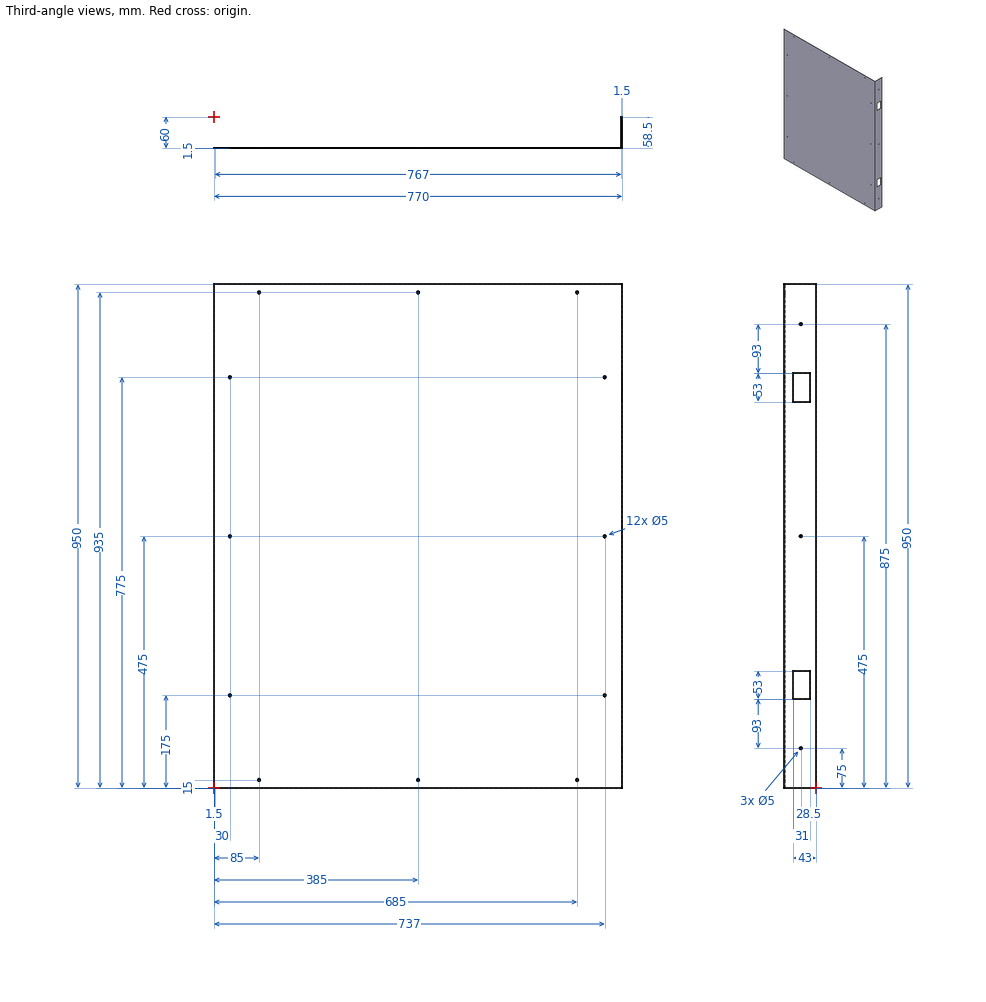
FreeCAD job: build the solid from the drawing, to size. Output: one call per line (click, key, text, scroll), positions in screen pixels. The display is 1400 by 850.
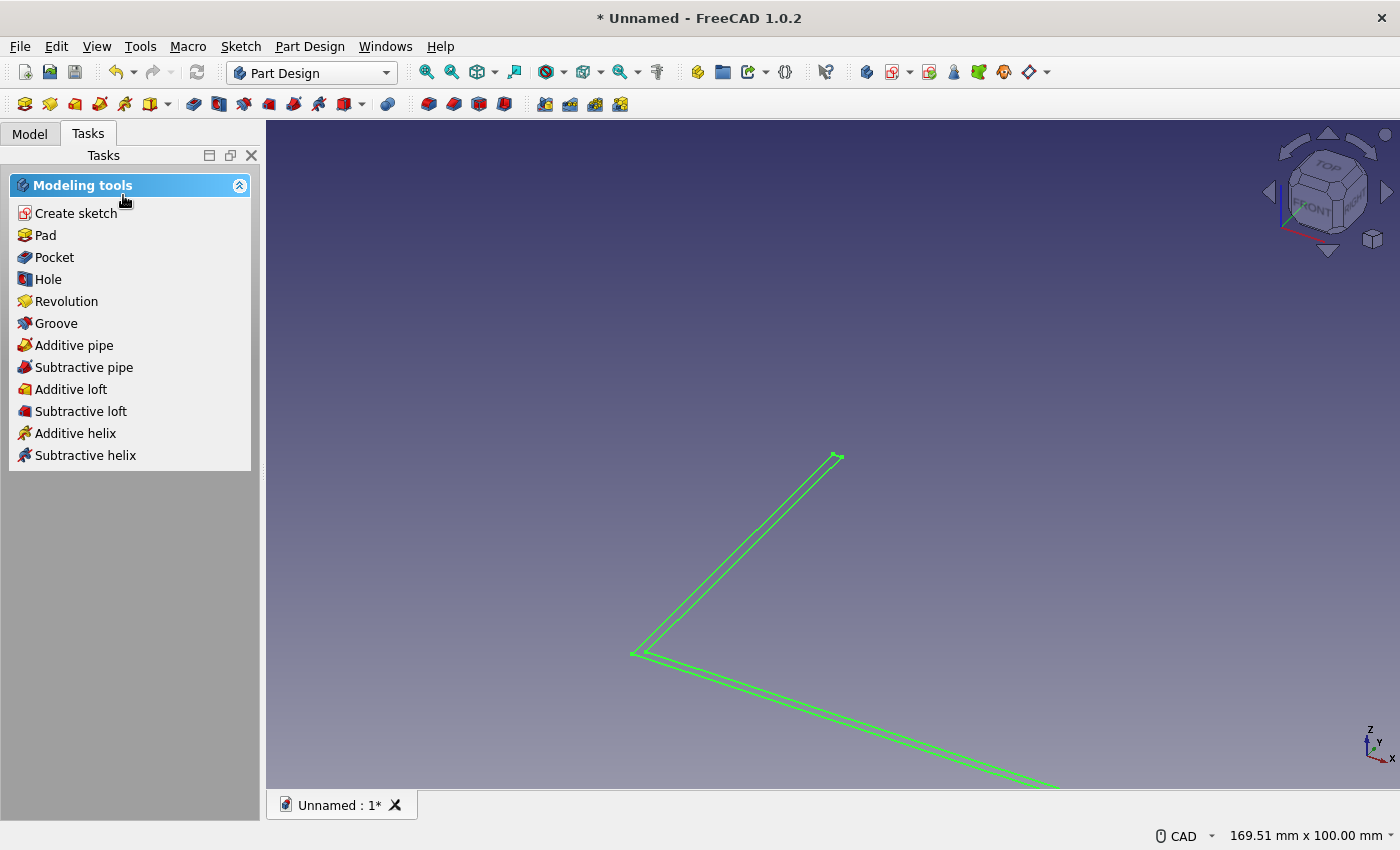
click(25, 104)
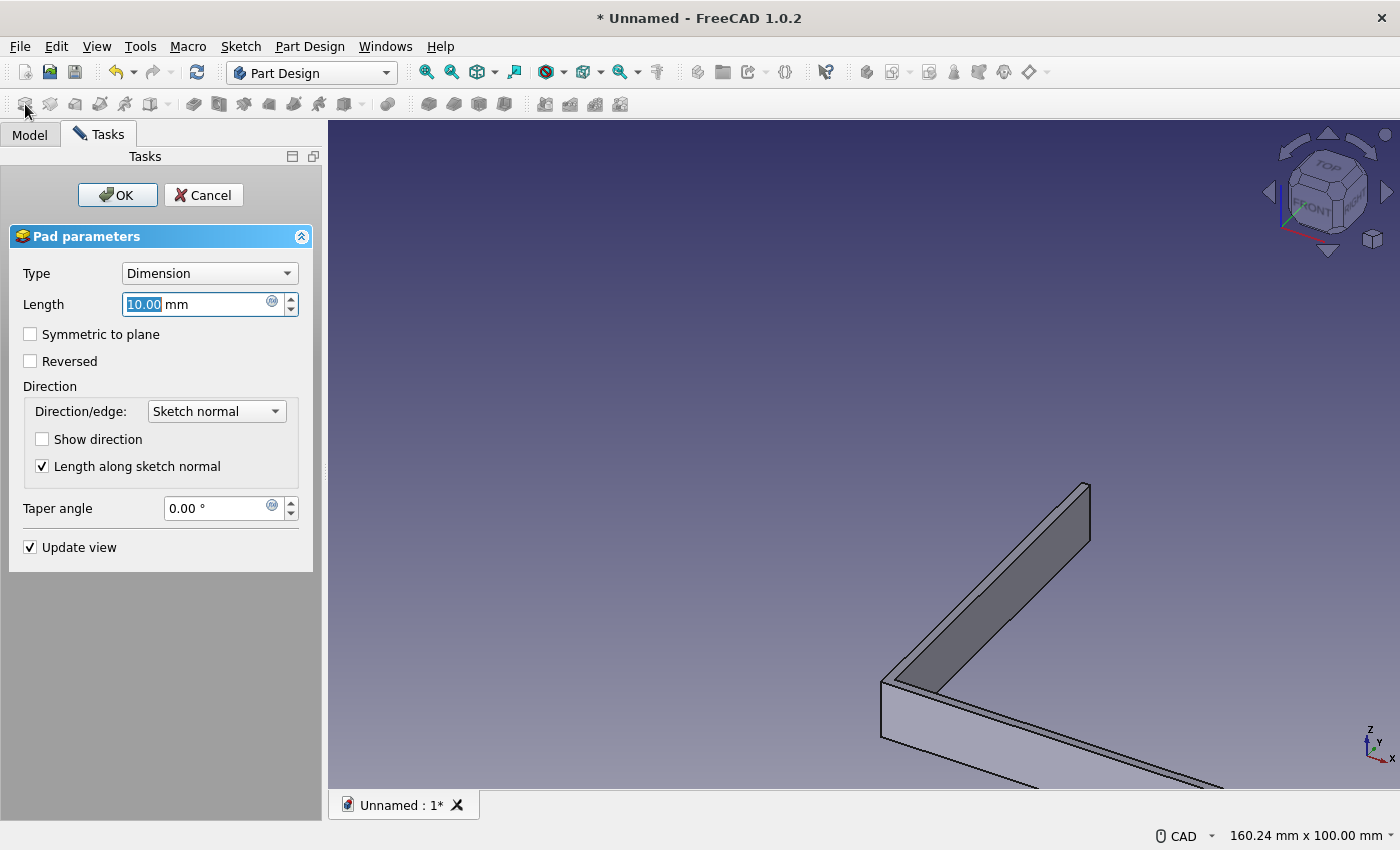
text(950)
key(Tab)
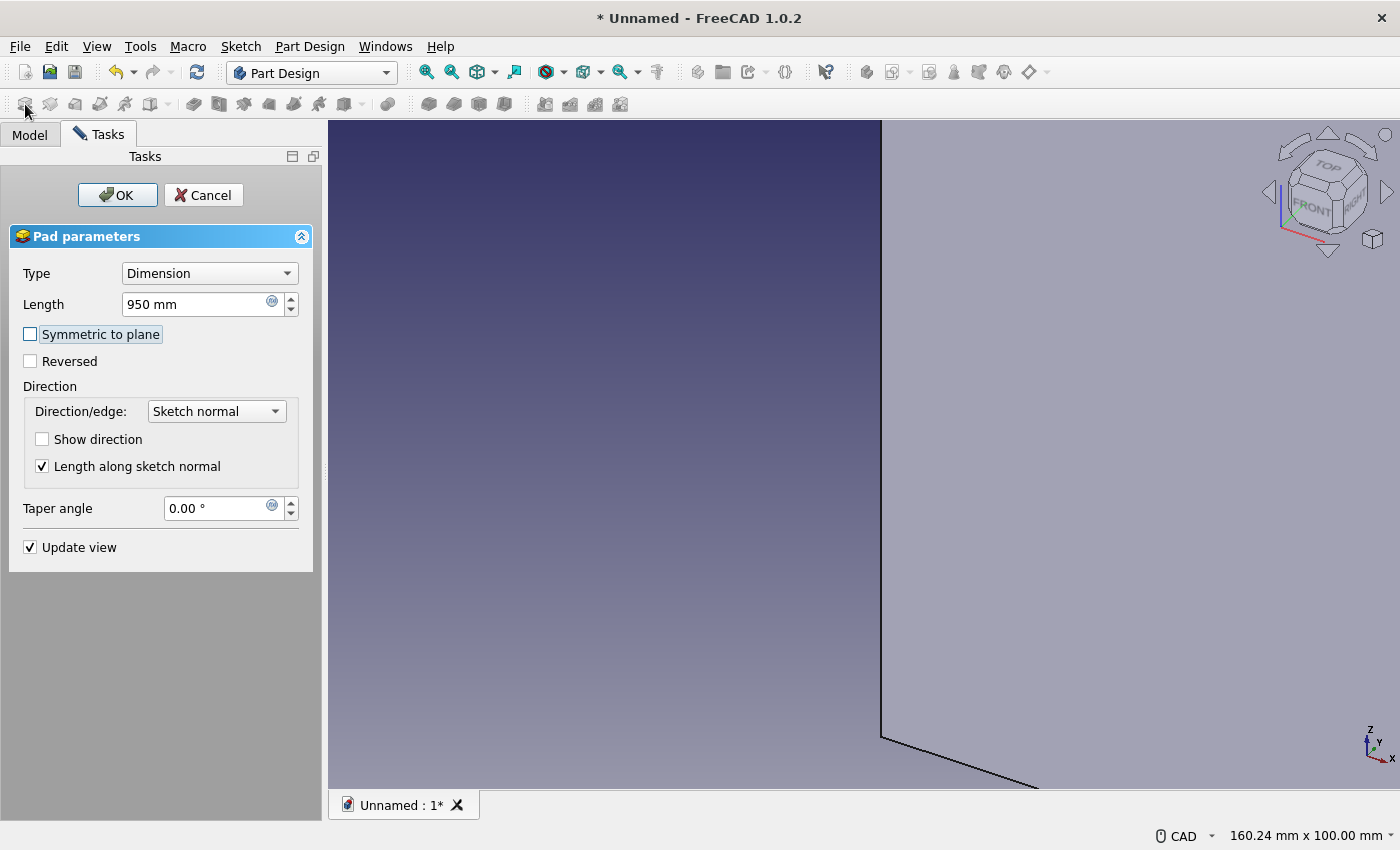
click(118, 195)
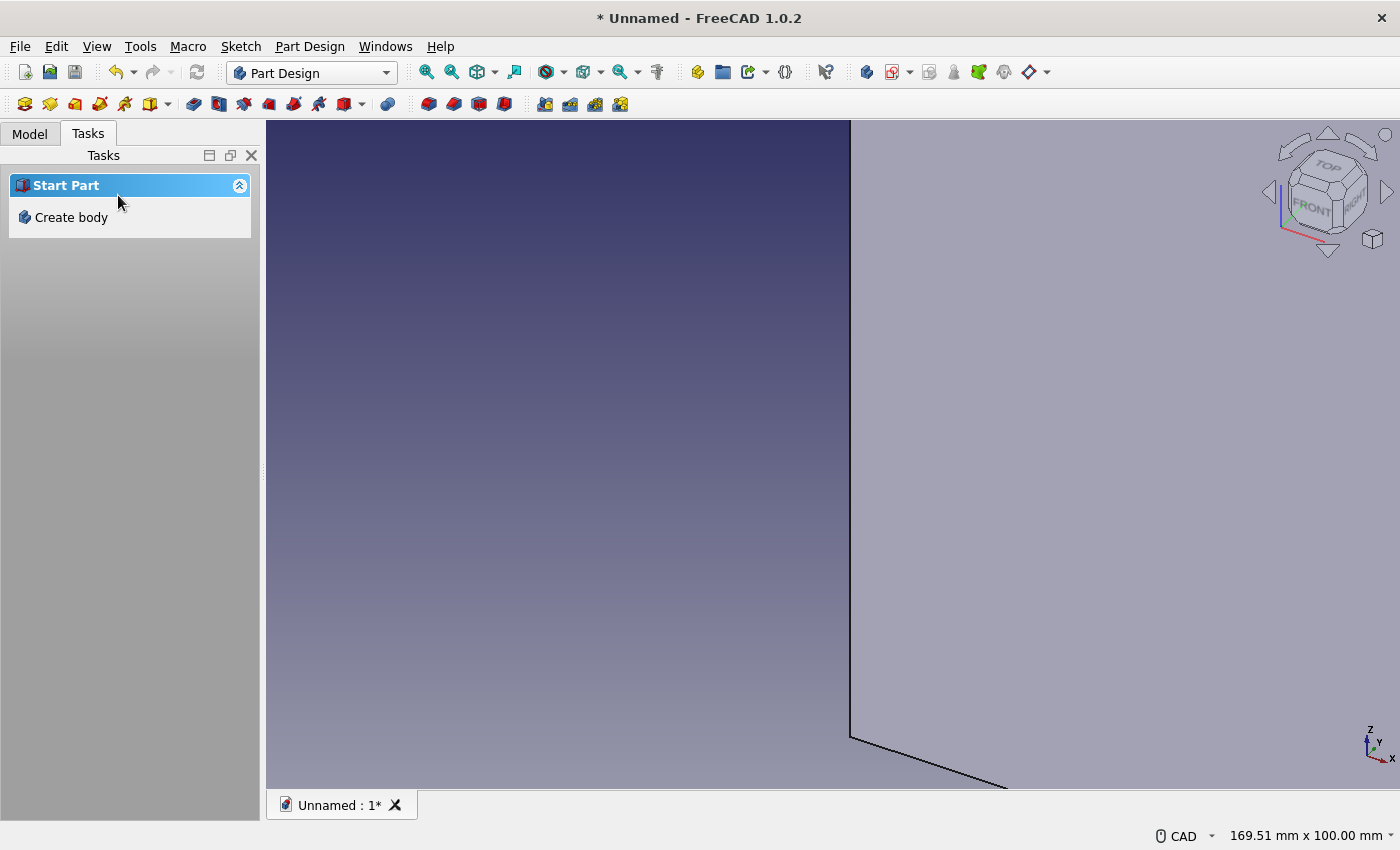
click(427, 72)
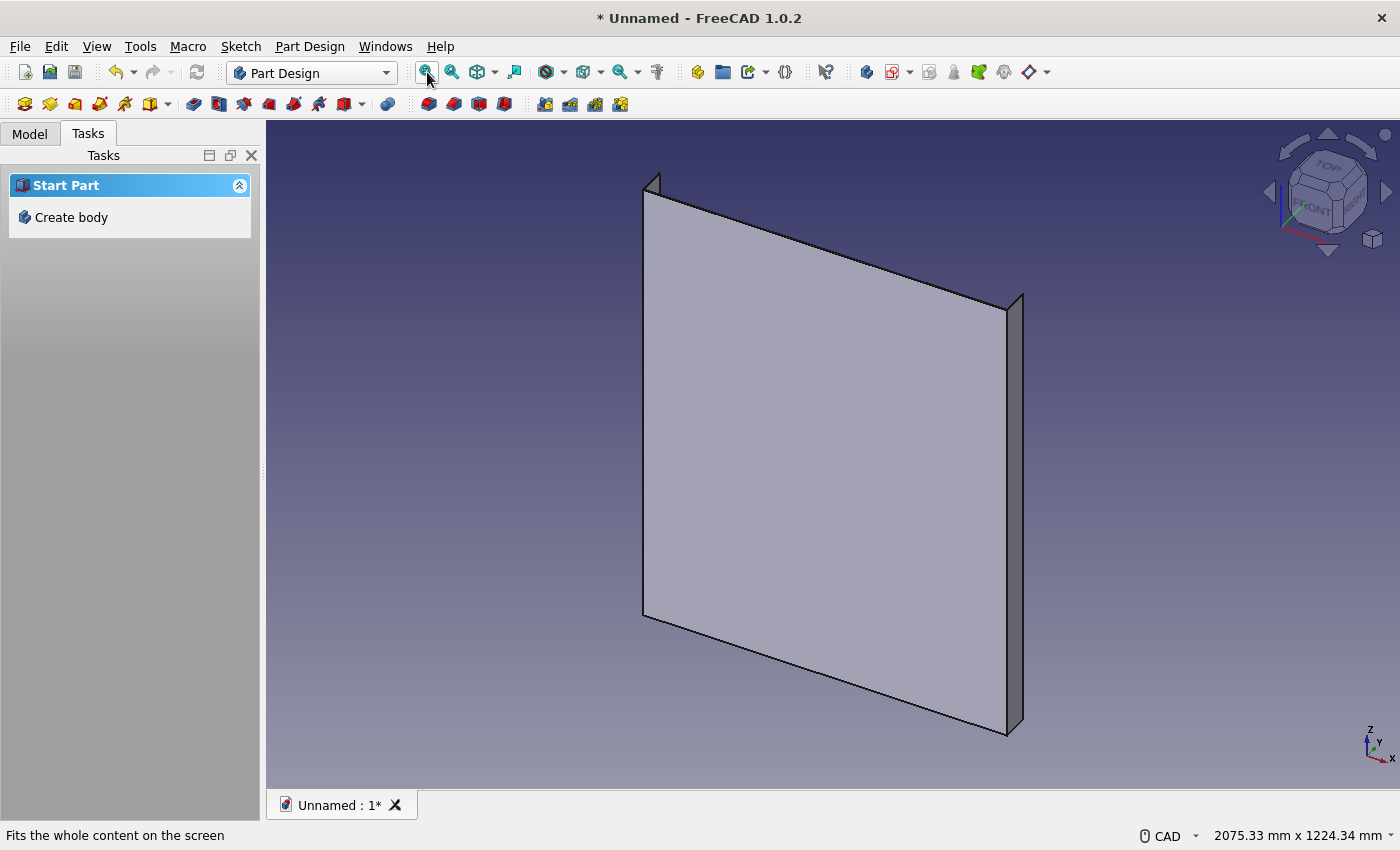
click(1015, 332)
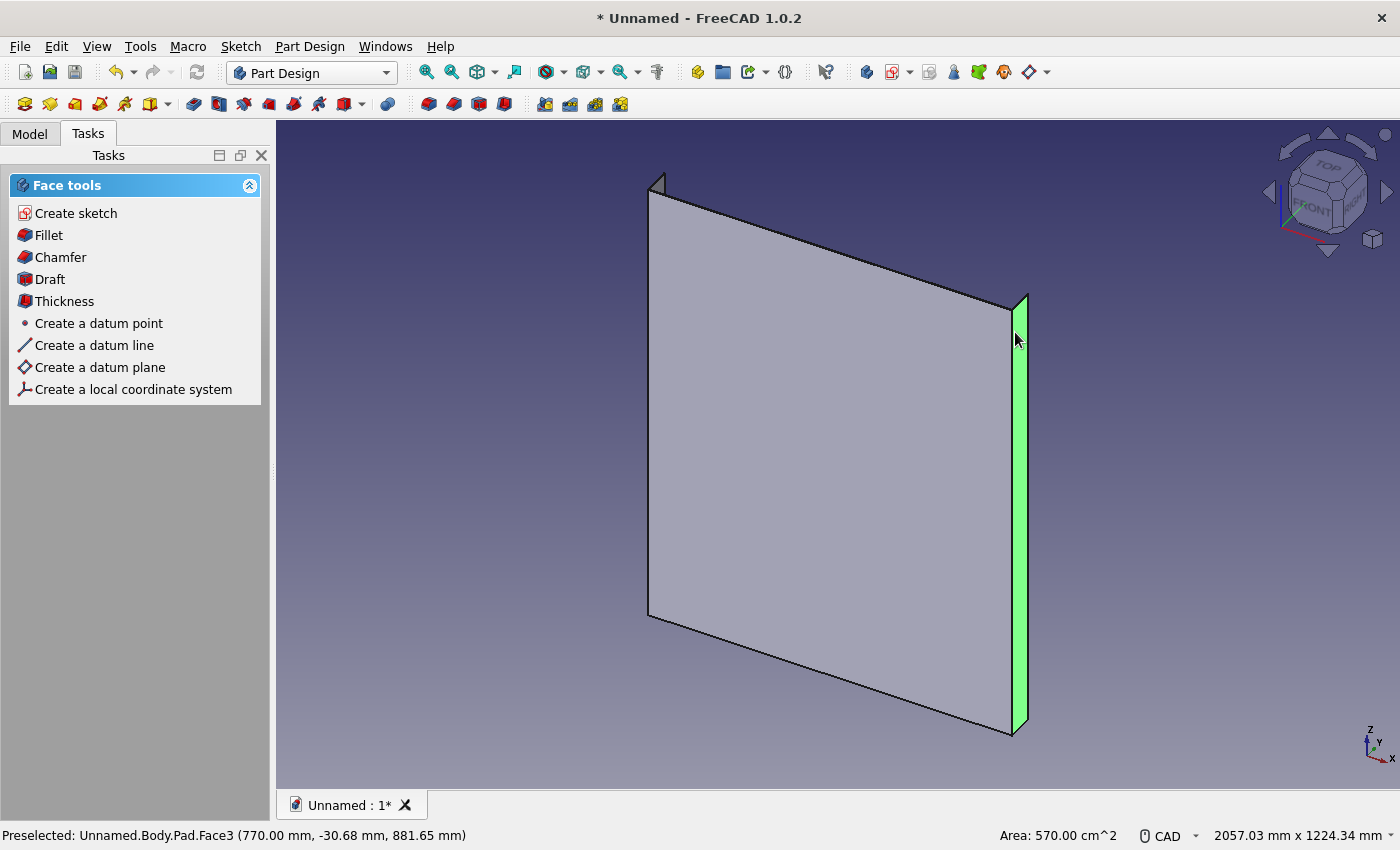
click(892, 72)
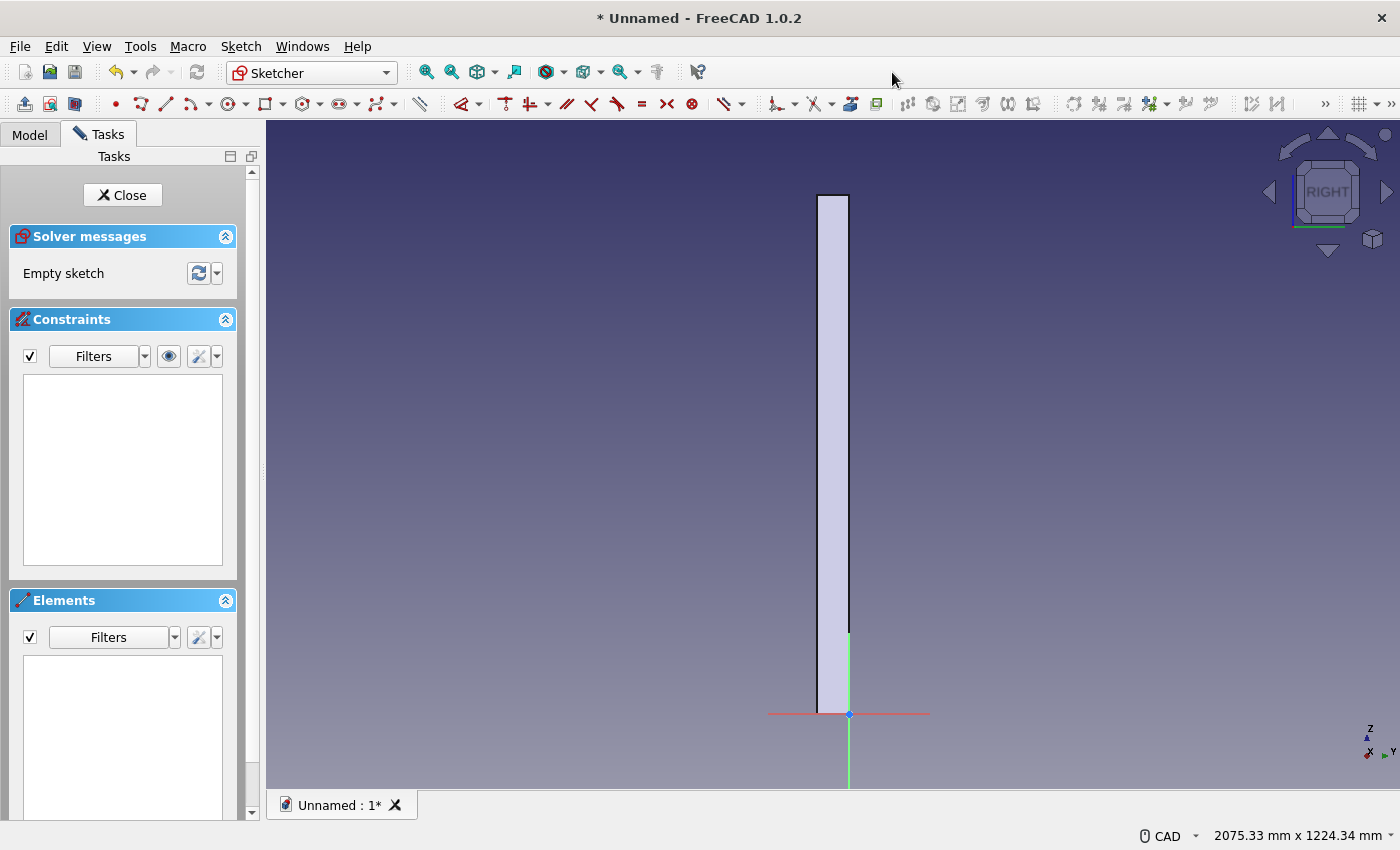
key(g)
key(r)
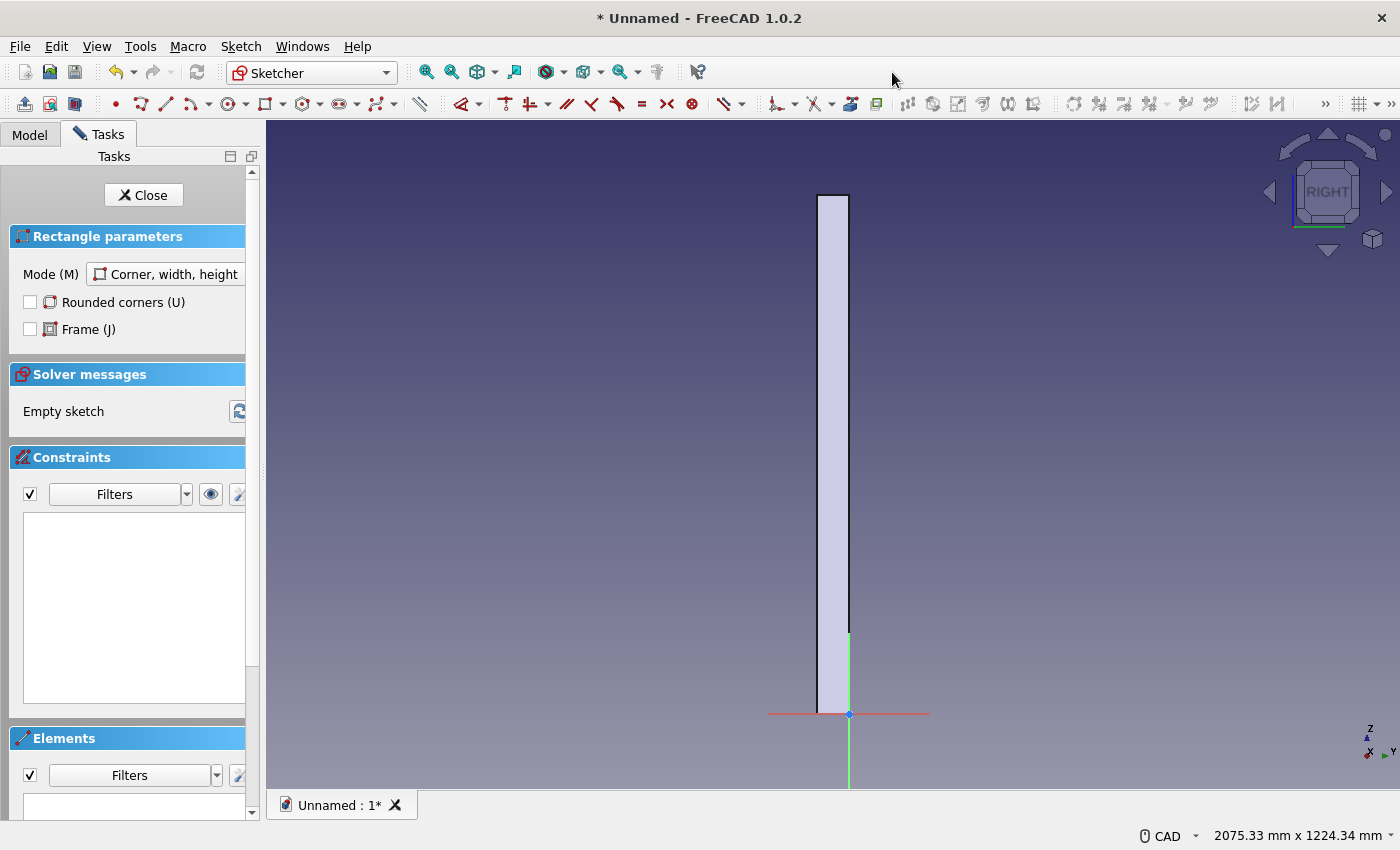
click(826, 593)